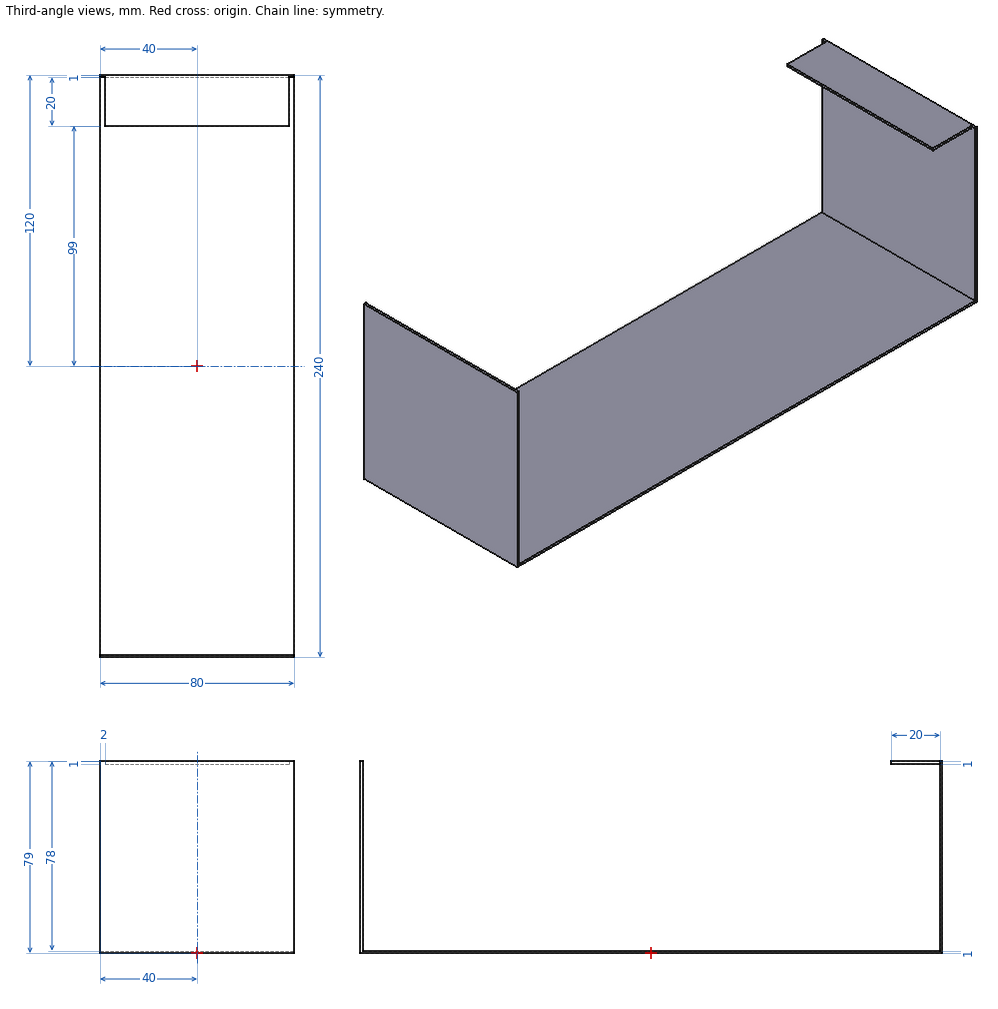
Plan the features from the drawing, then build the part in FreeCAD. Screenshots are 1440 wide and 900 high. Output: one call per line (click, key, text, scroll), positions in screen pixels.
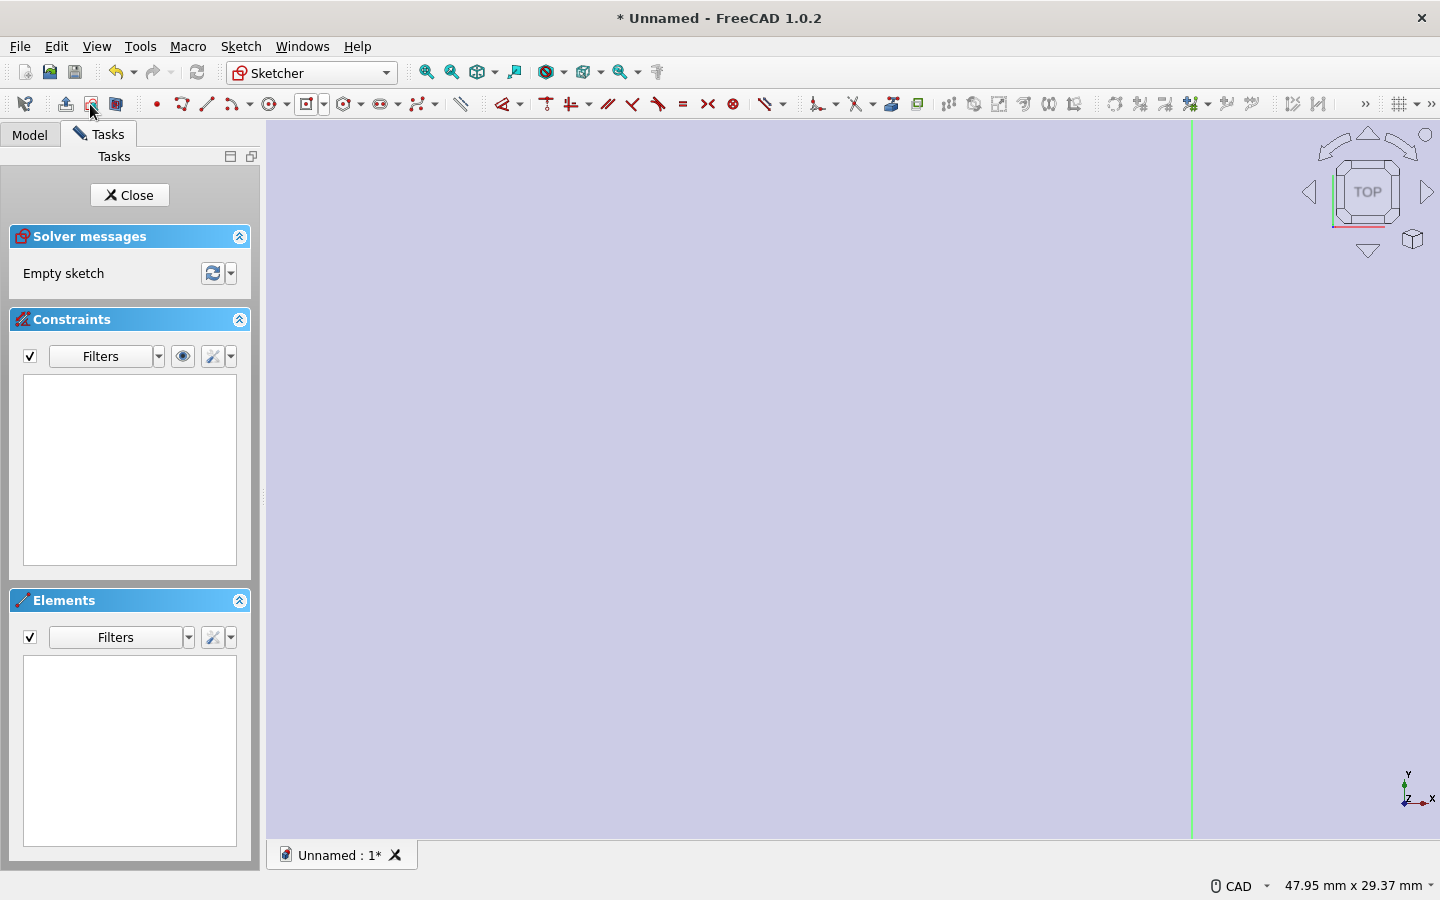
scroll(721, 811, down, 10)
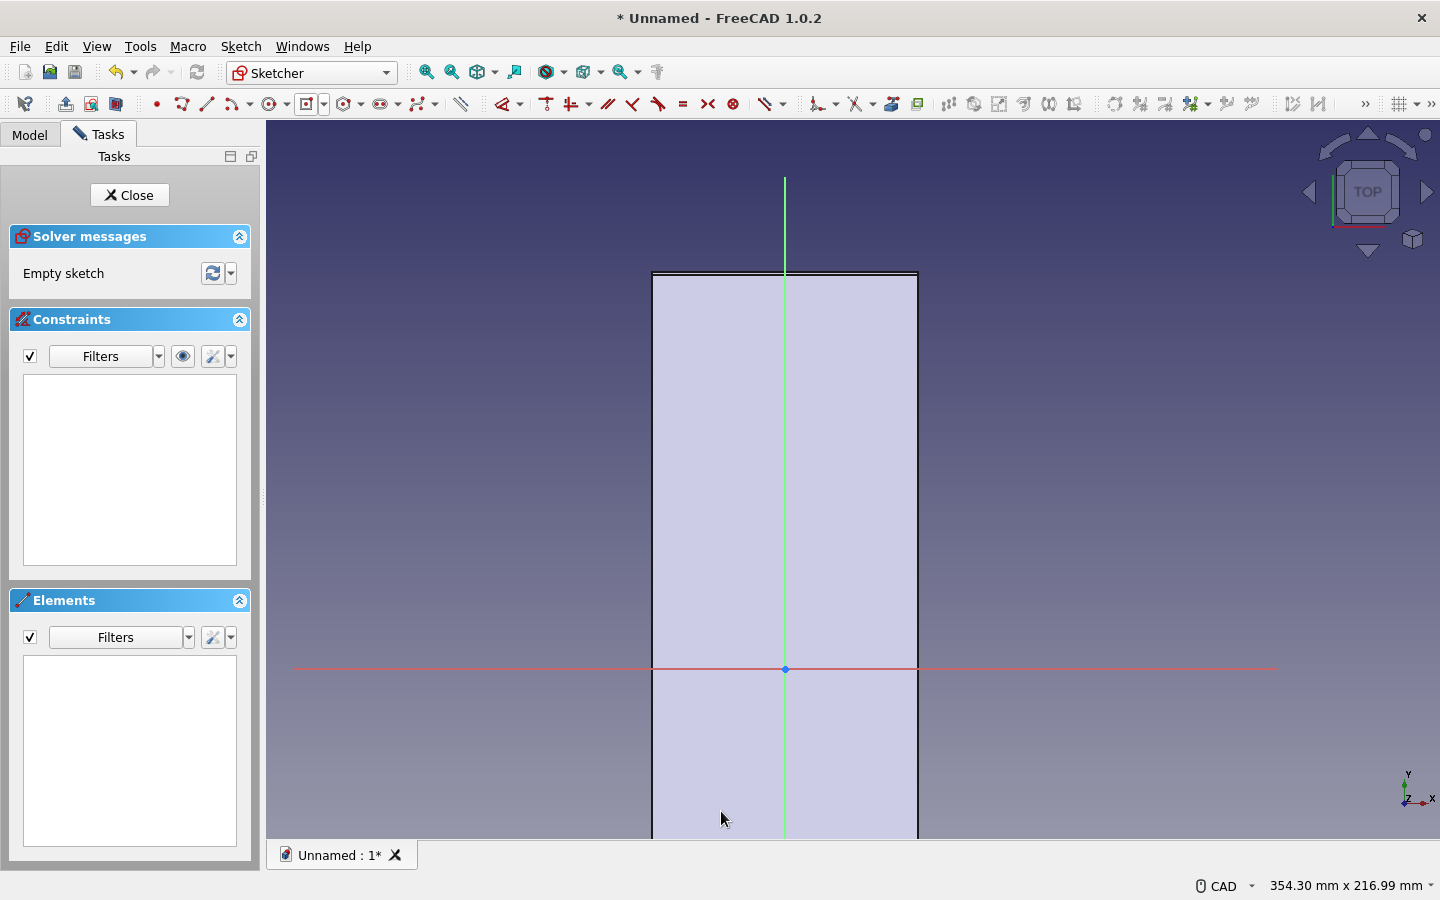
click(324, 104)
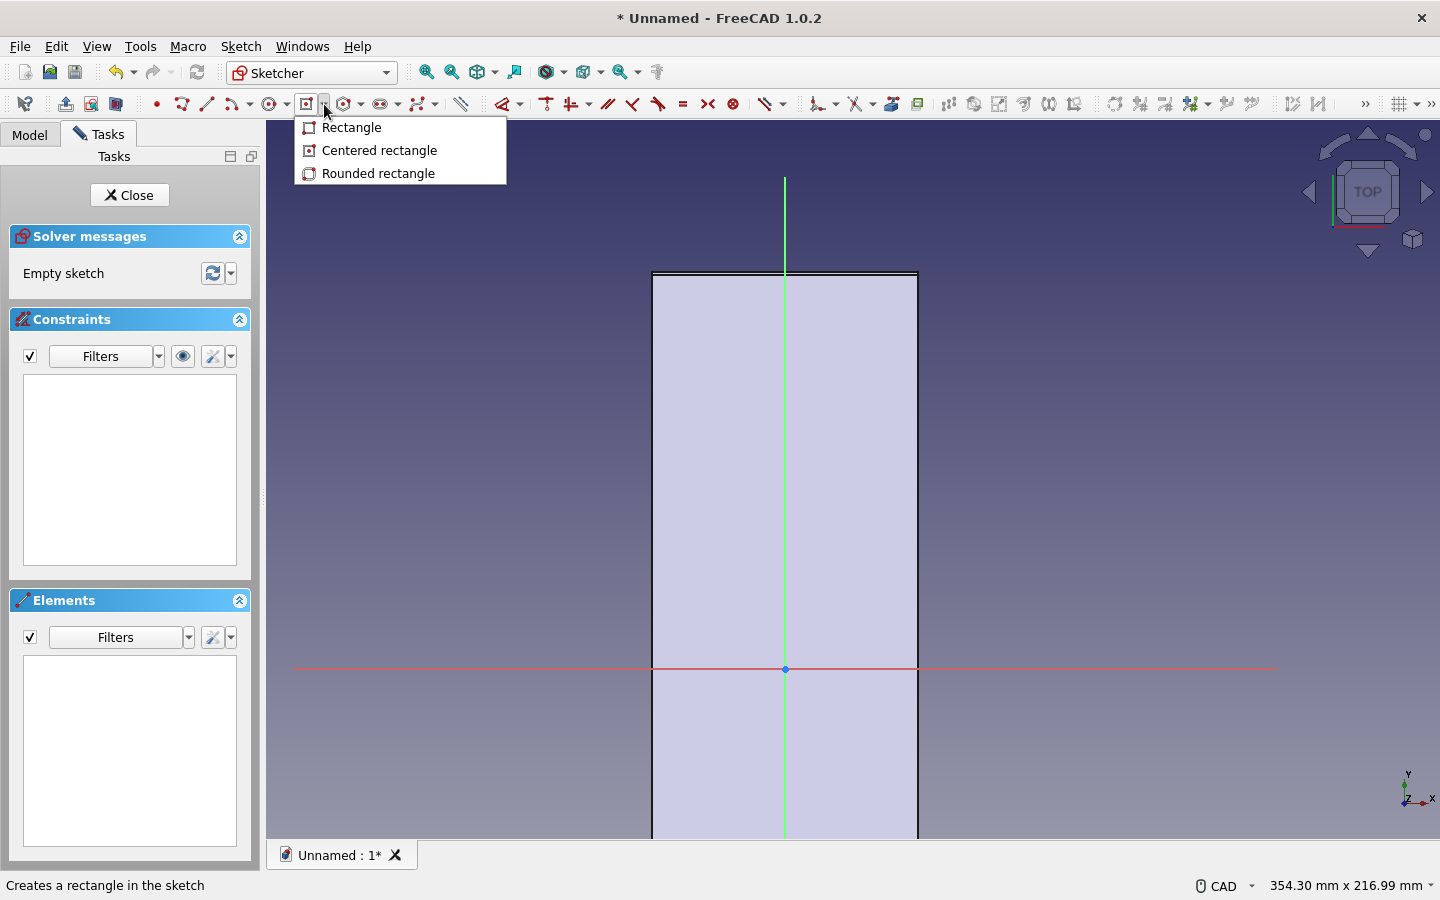
click(400, 128)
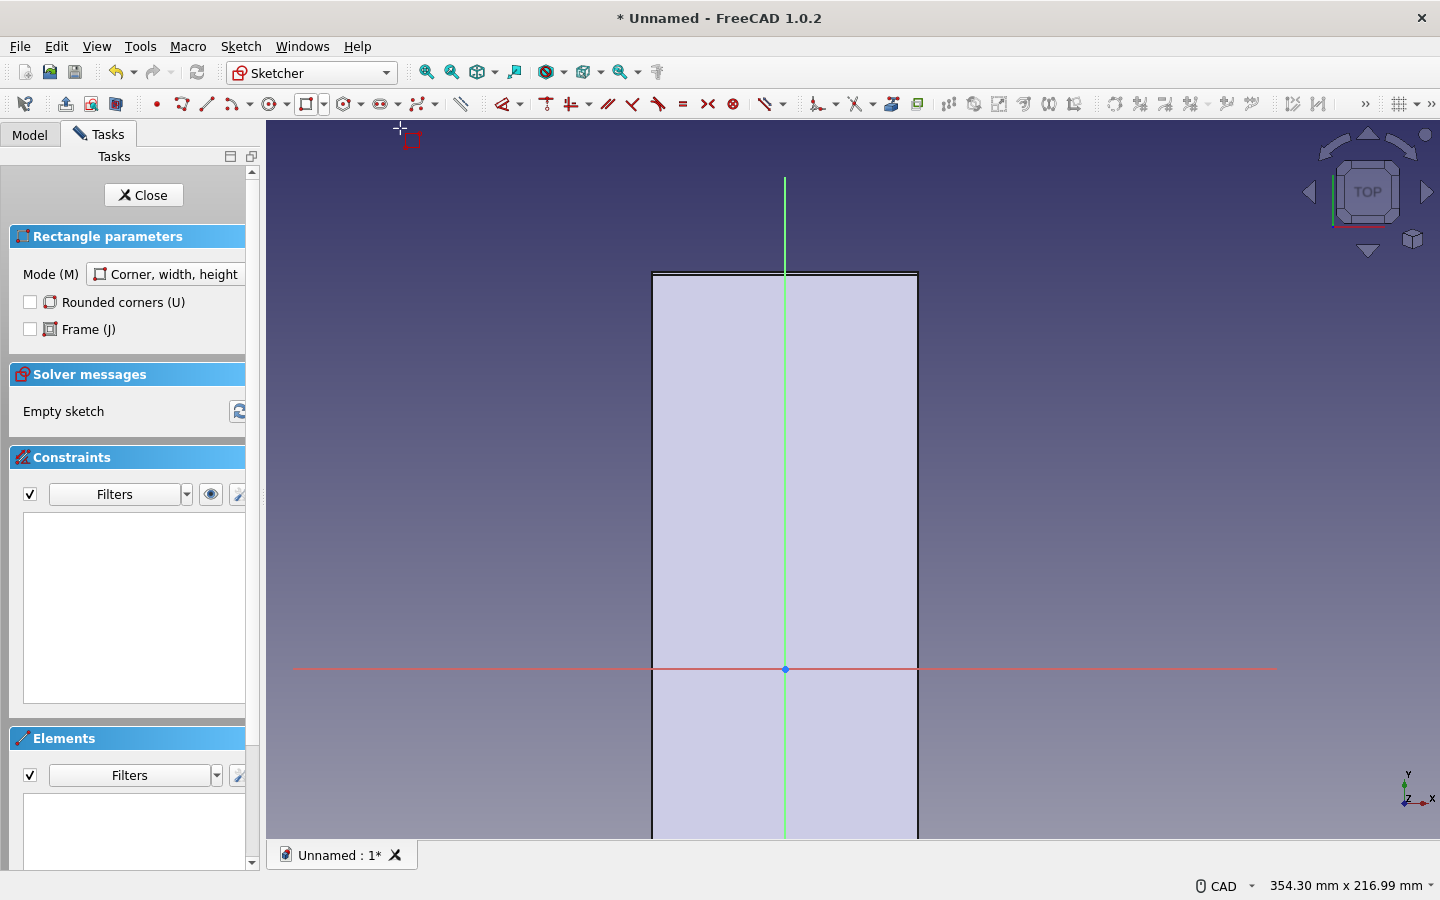
click(653, 275)
click(918, 341)
key(Escape)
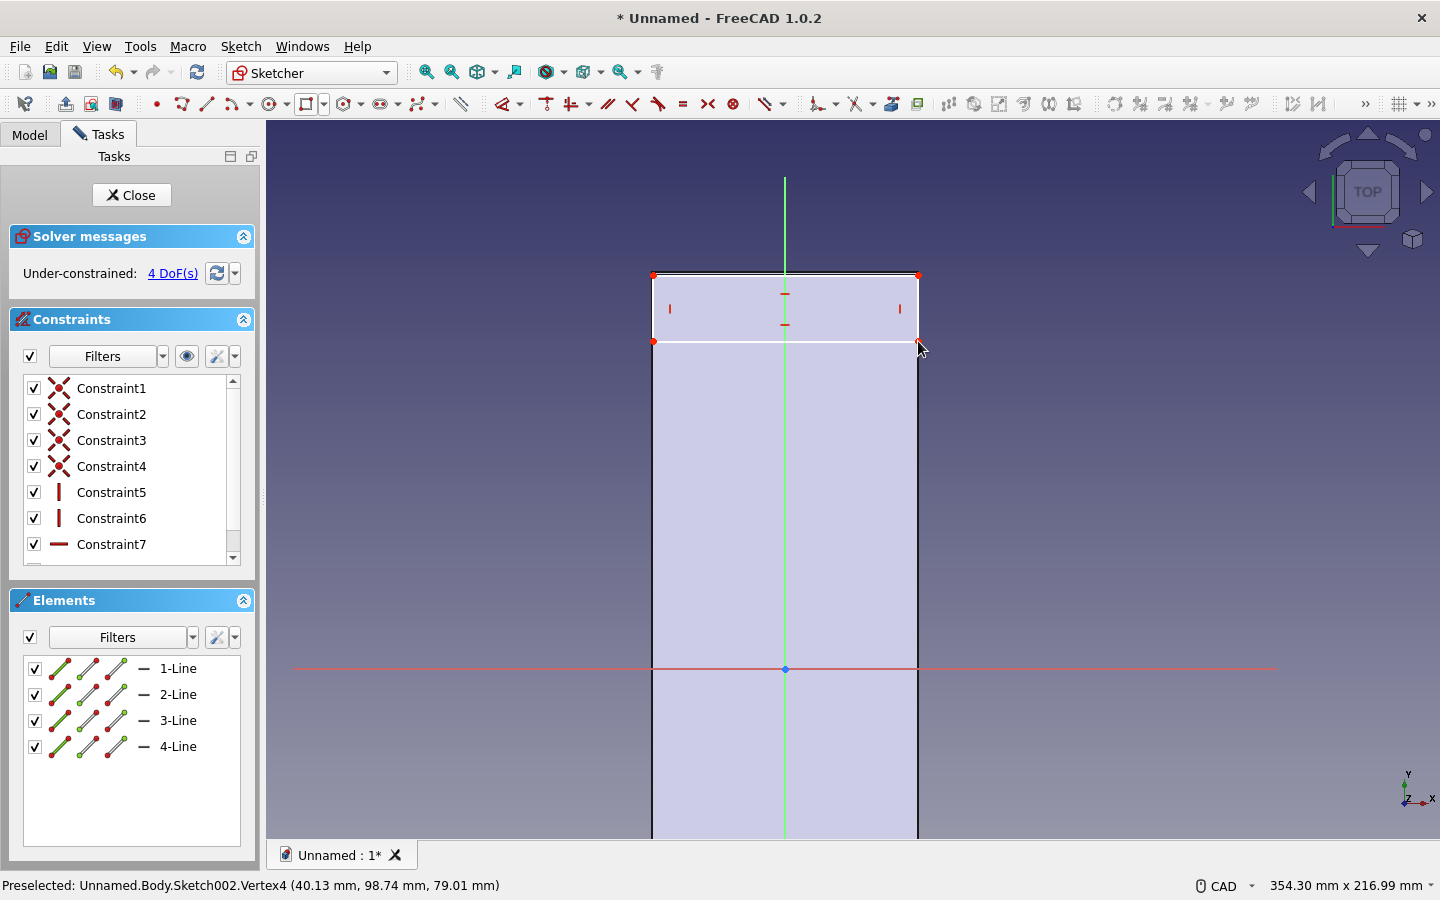
click(502, 104)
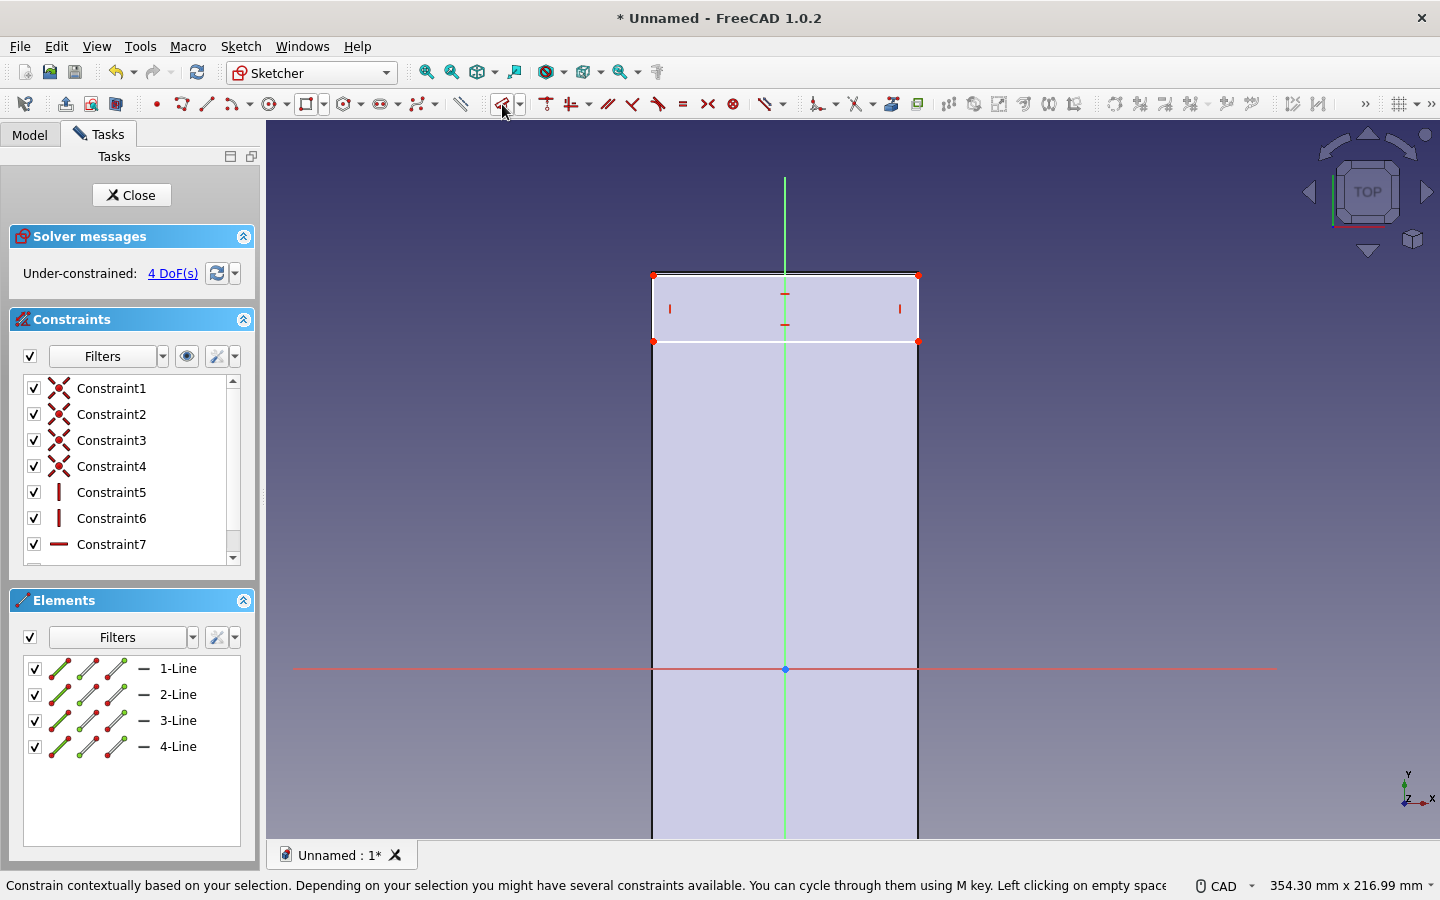
click(653, 296)
click(619, 309)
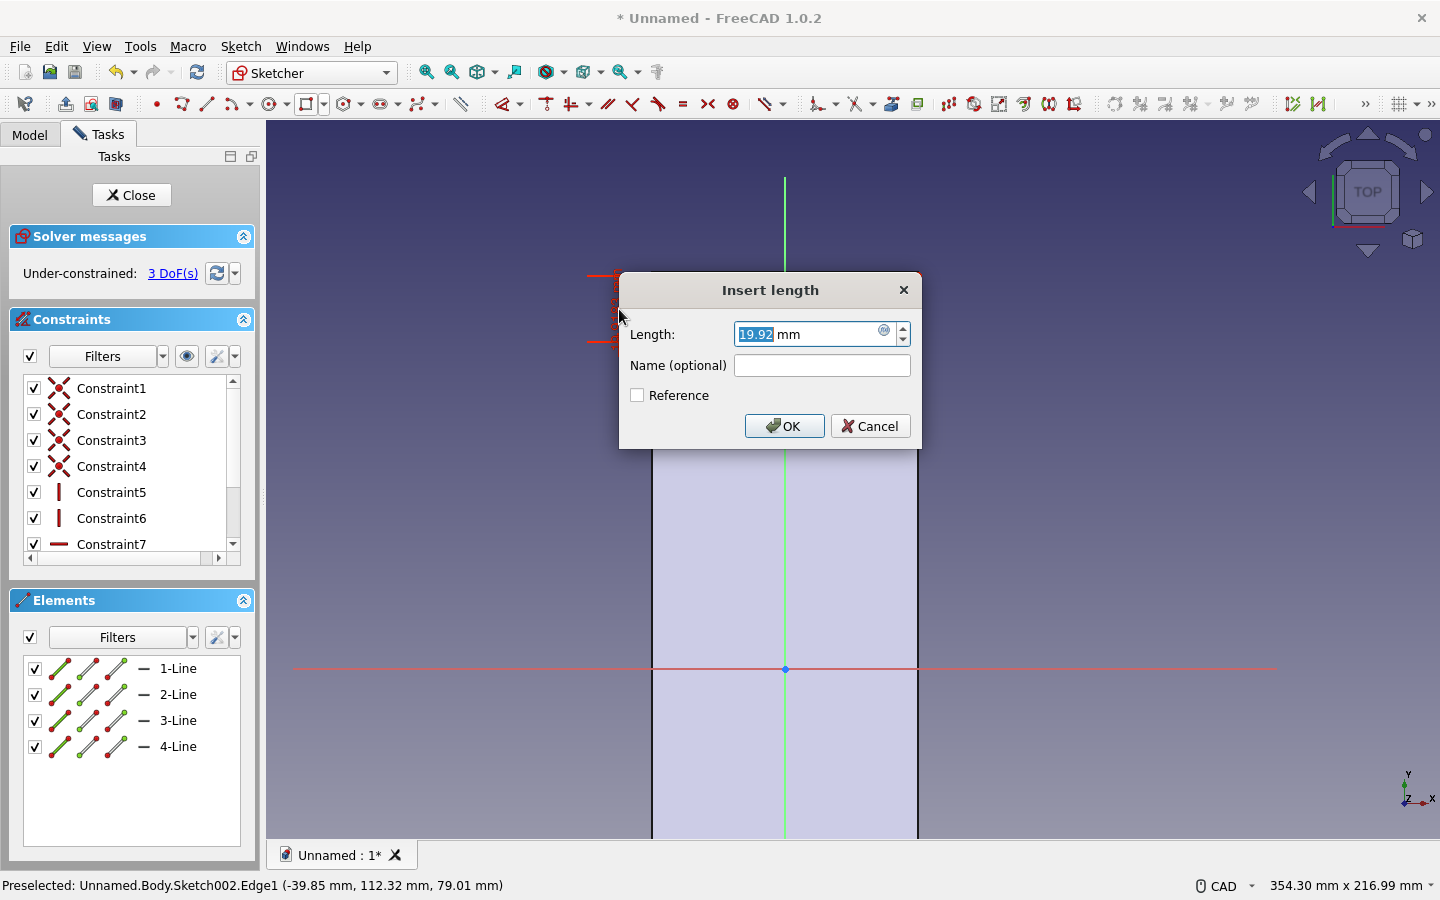
text(20)
key(Return)